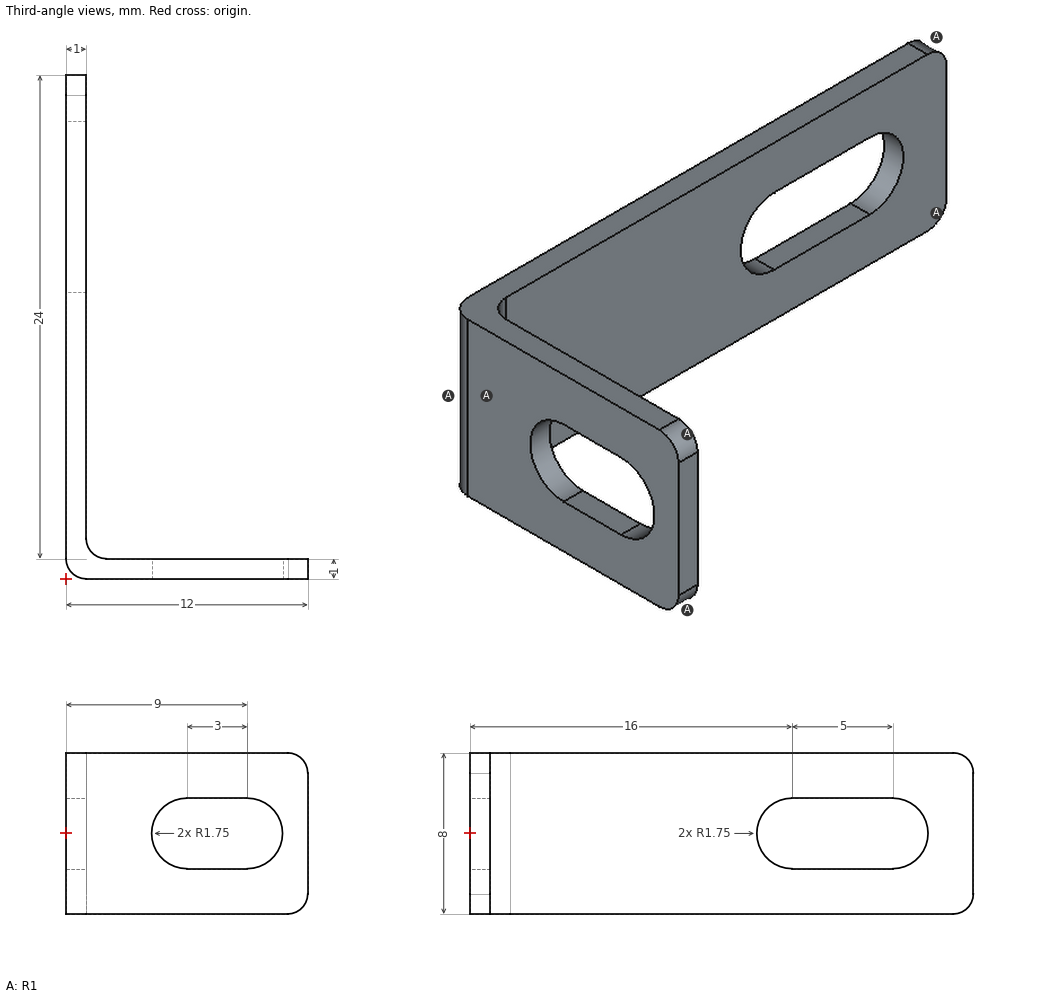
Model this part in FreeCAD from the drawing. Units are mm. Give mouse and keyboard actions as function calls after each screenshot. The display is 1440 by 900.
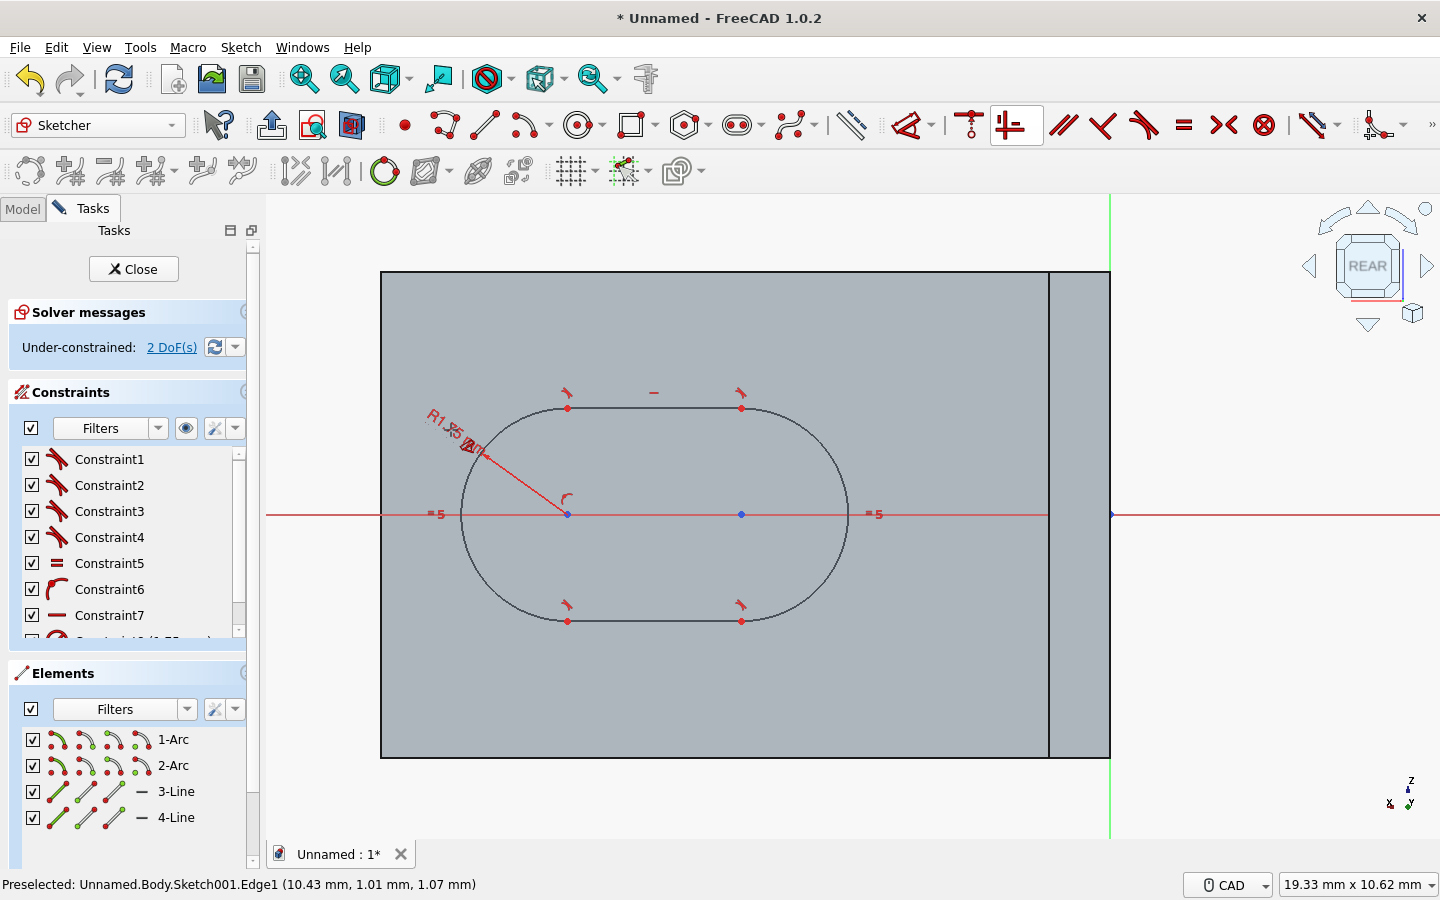
click(620, 408)
click(655, 374)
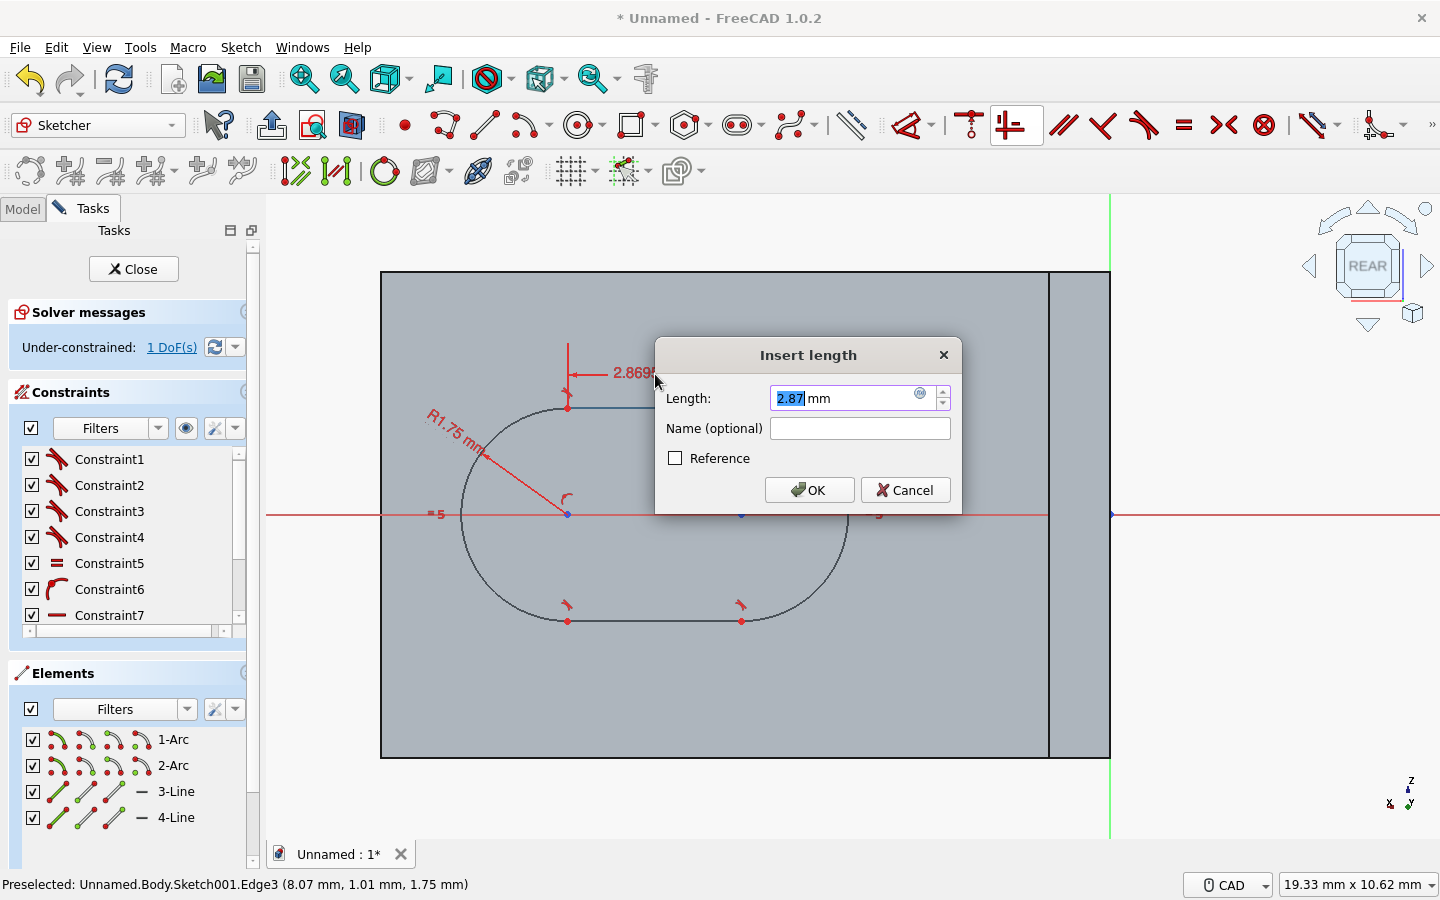
text(3)
key(Return)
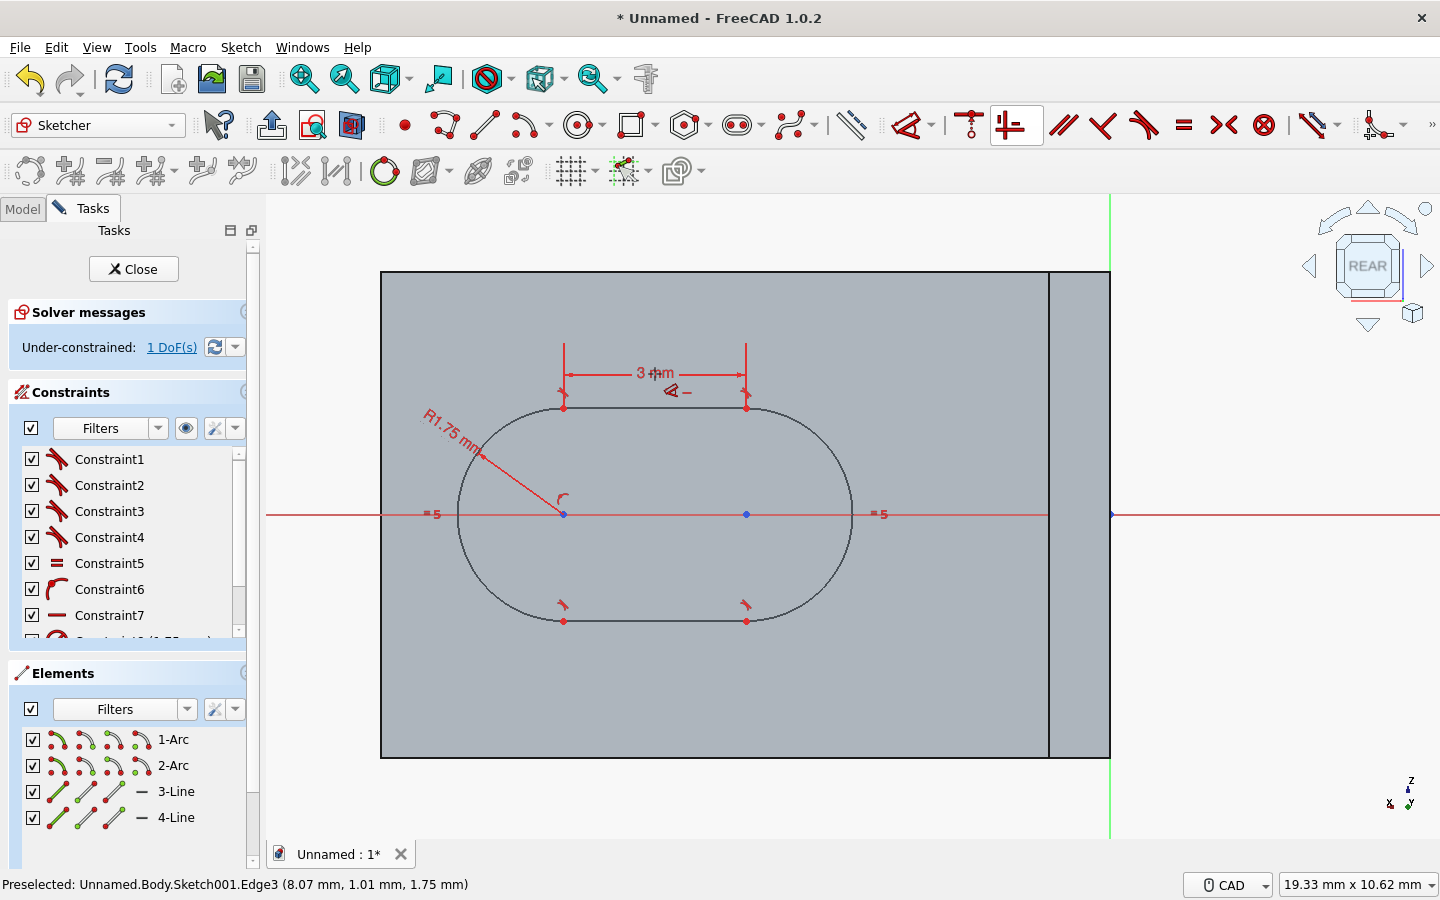
click(564, 408)
click(837, 374)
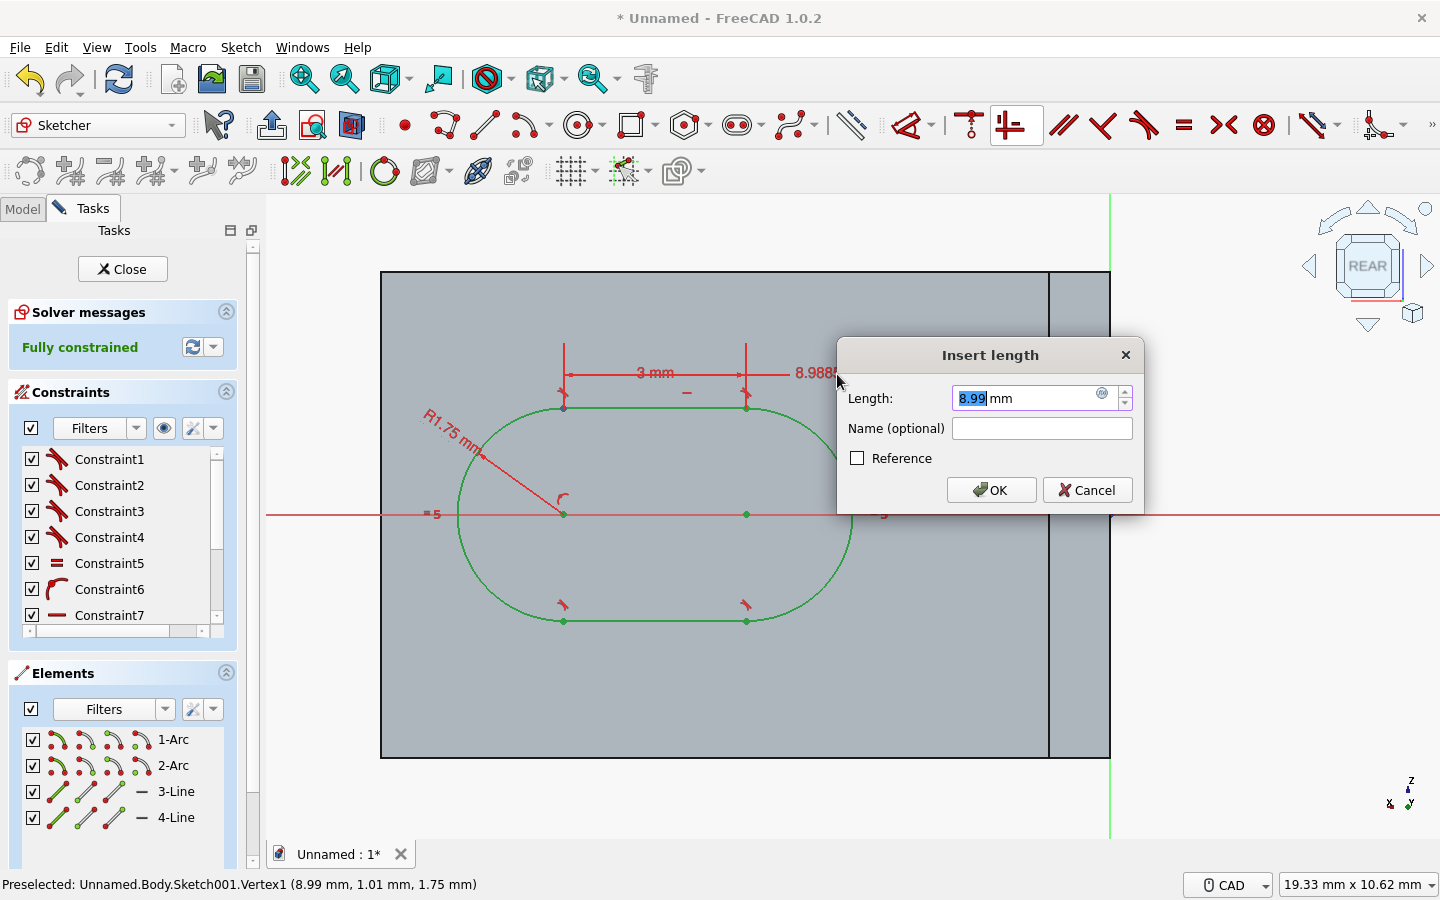
text(9)
key(Return)
key(Escape)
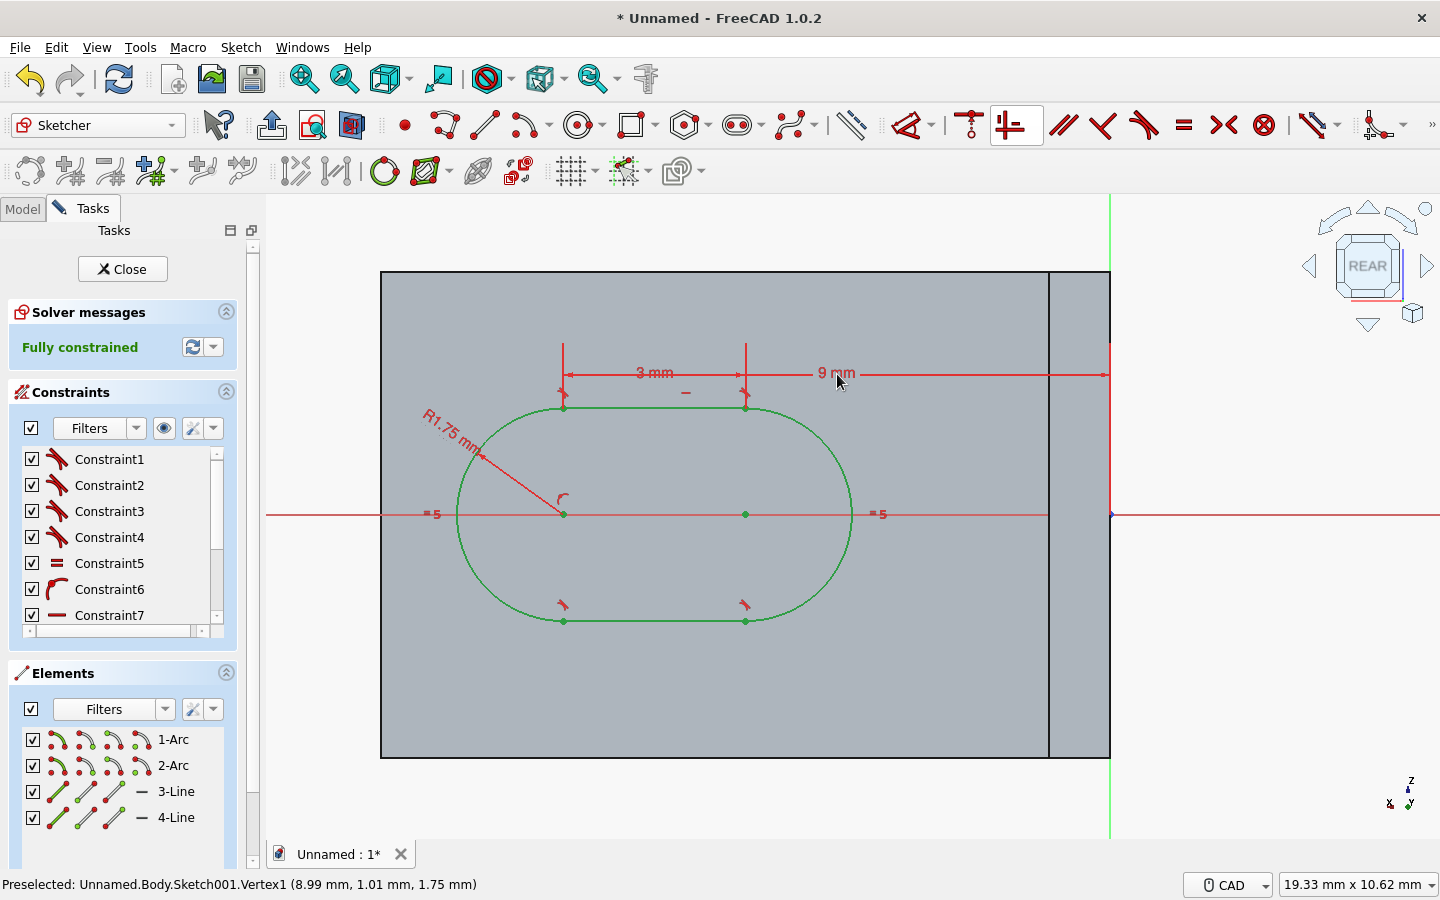
click(123, 269)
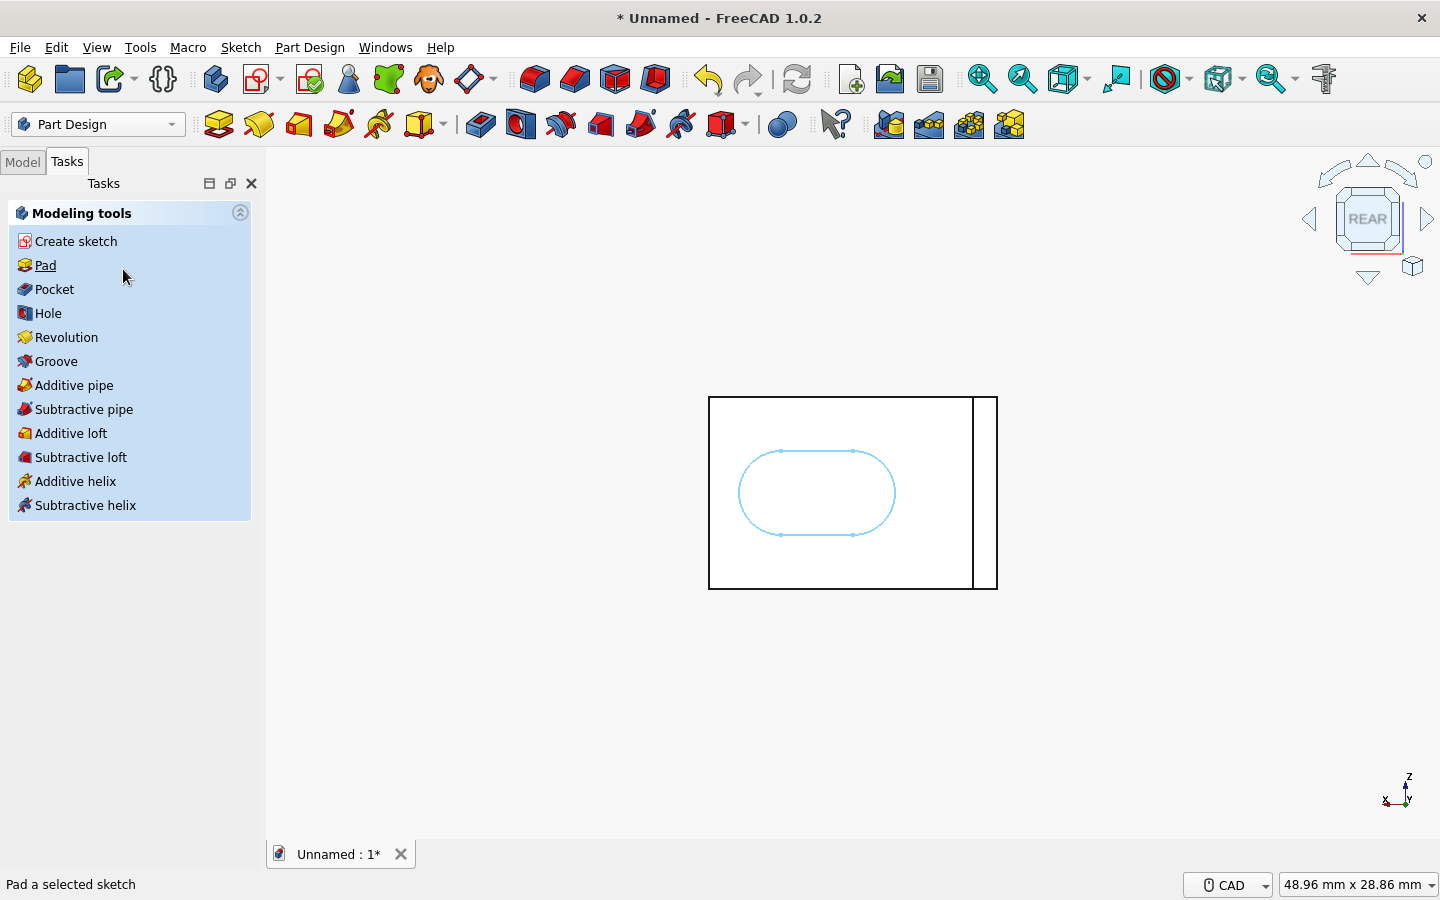
click(482, 124)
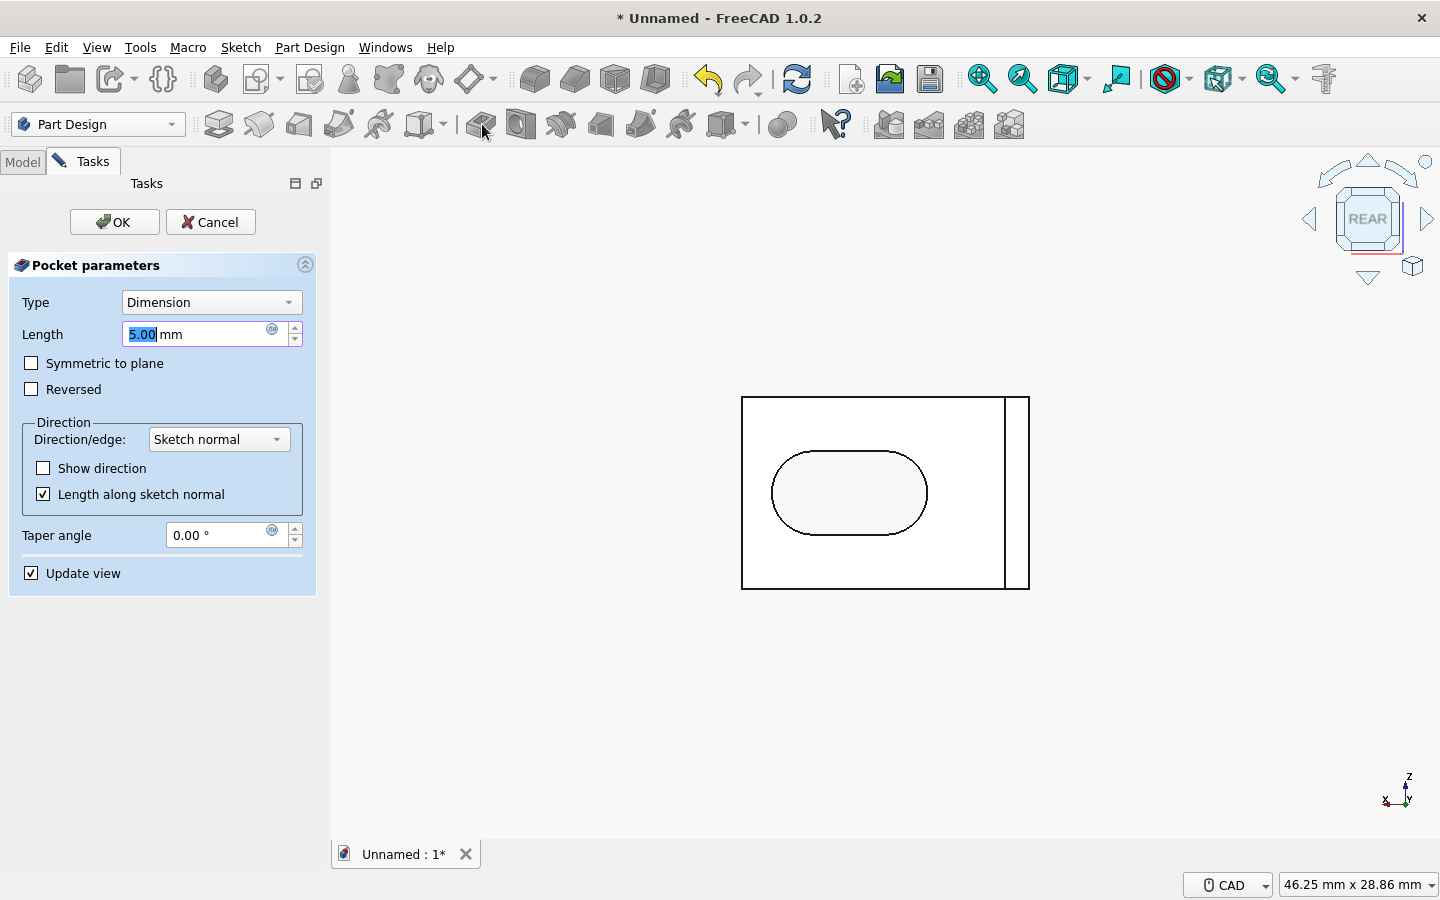
click(212, 302)